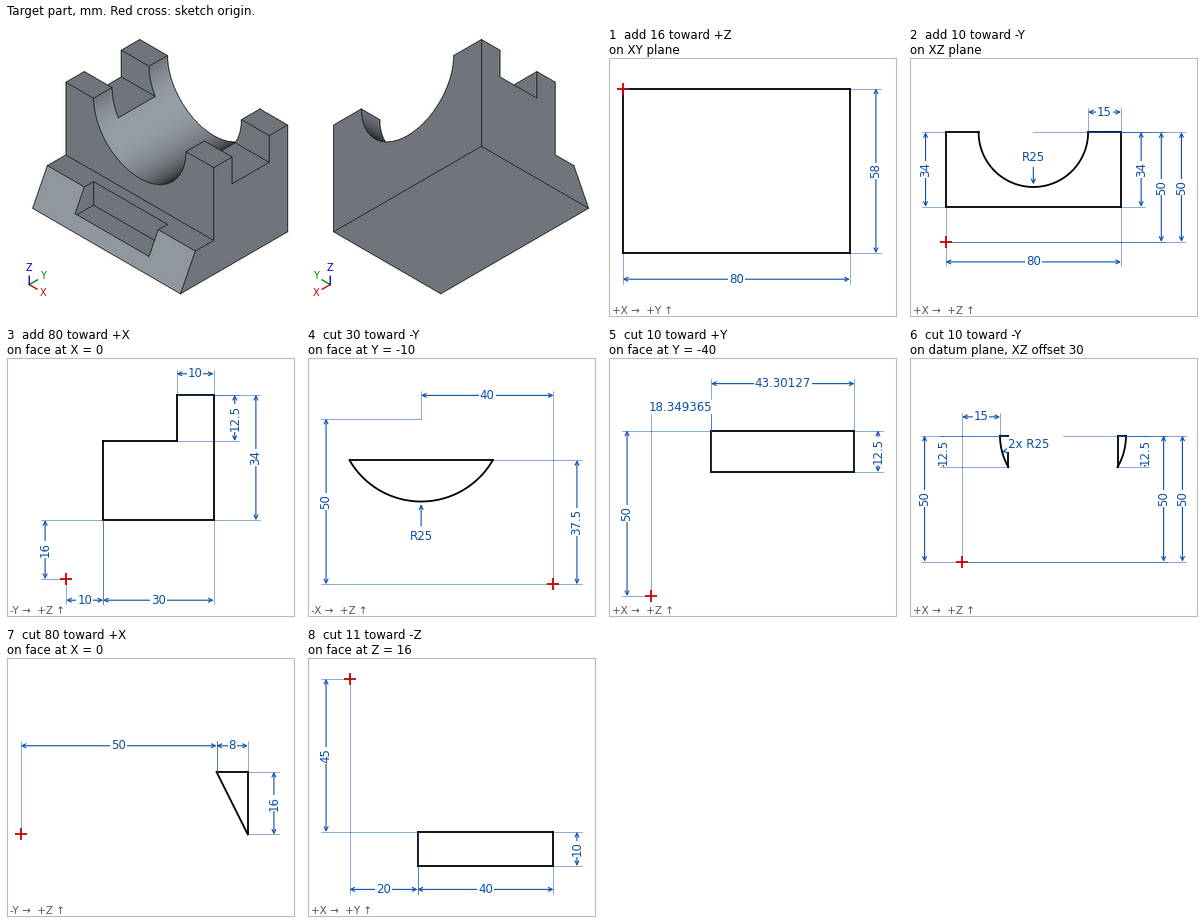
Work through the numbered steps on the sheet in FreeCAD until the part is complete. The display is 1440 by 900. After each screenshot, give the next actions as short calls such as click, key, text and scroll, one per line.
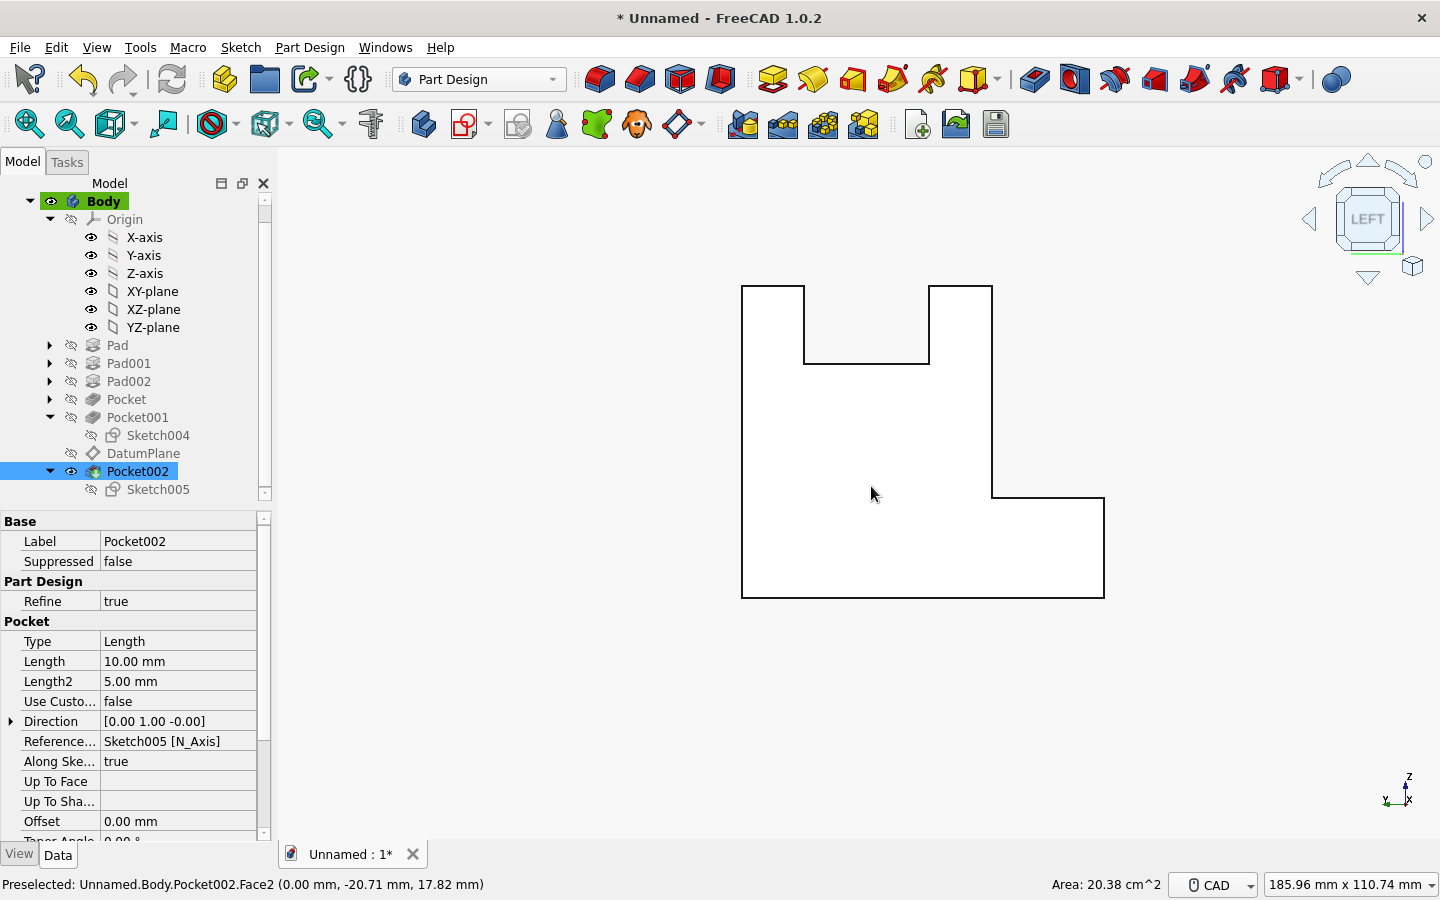
click(464, 124)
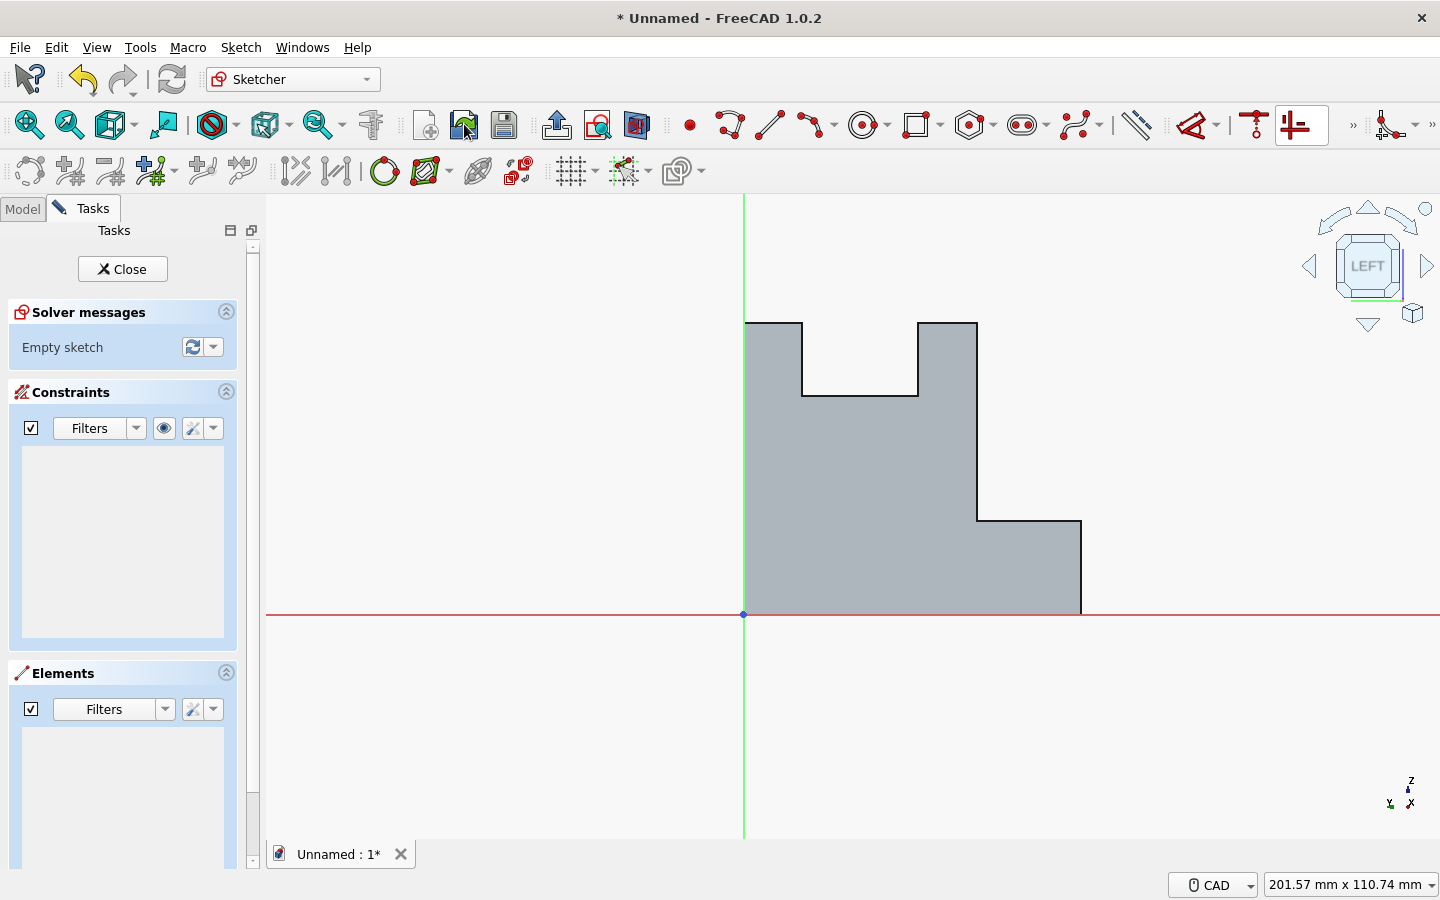
scroll(1148, 585, up, 7)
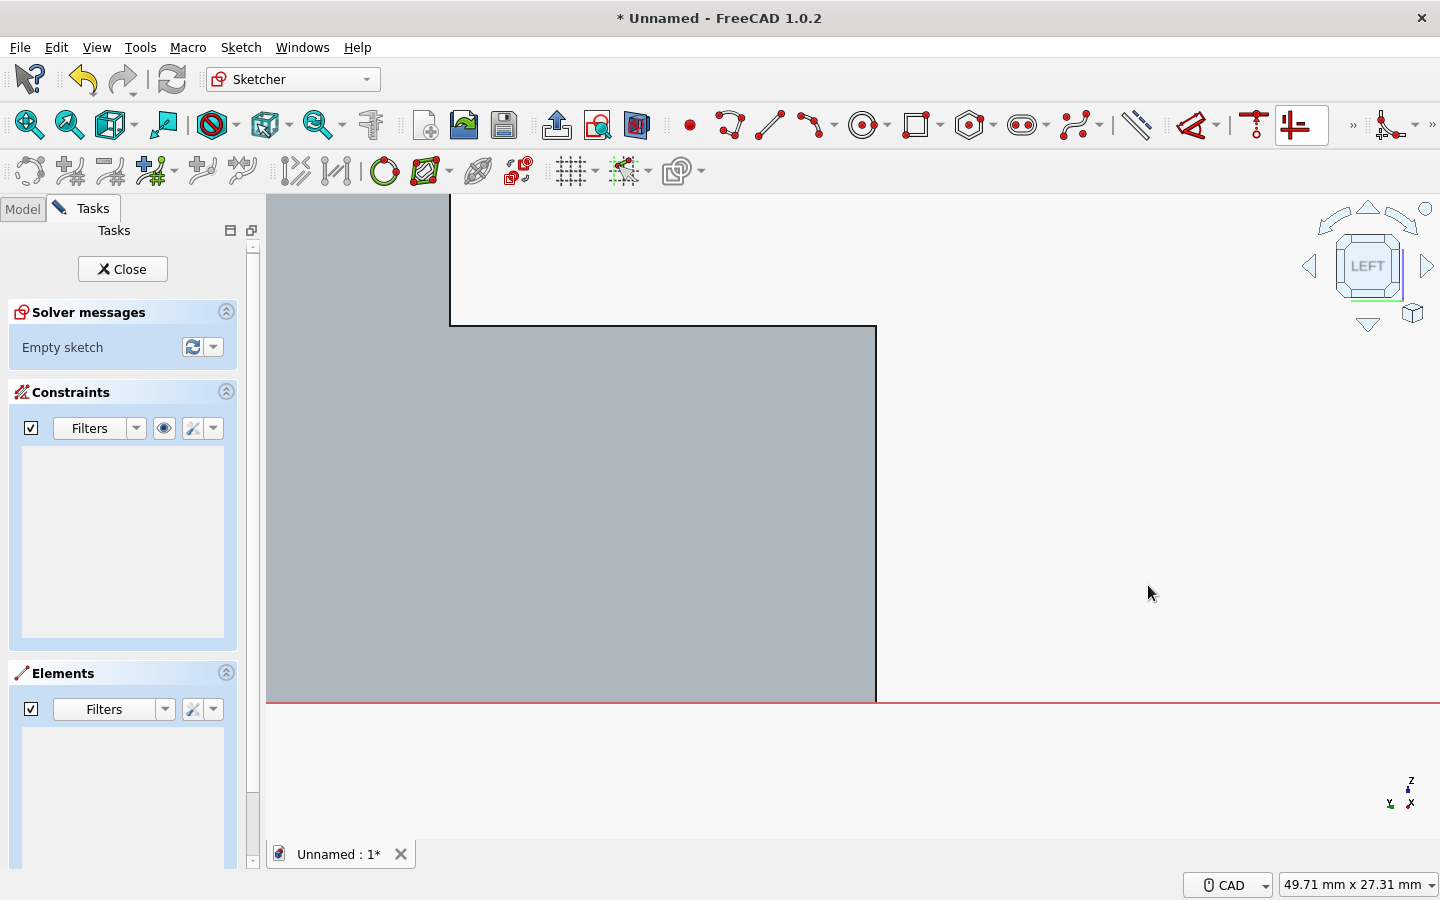
click(730, 126)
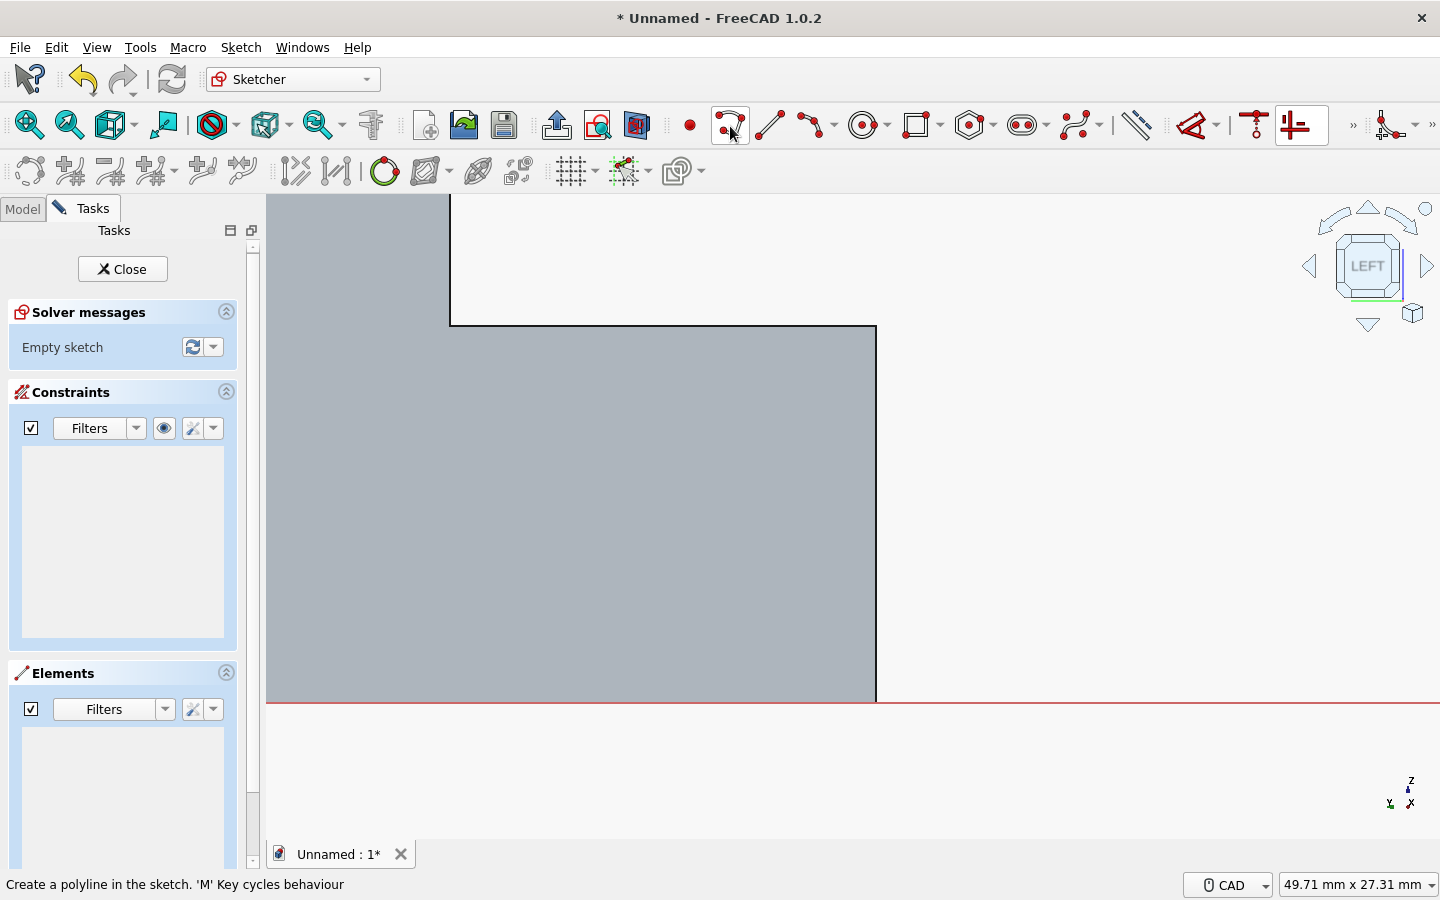
click(687, 326)
click(876, 703)
click(876, 326)
click(687, 327)
key(Escape)
key(Escape)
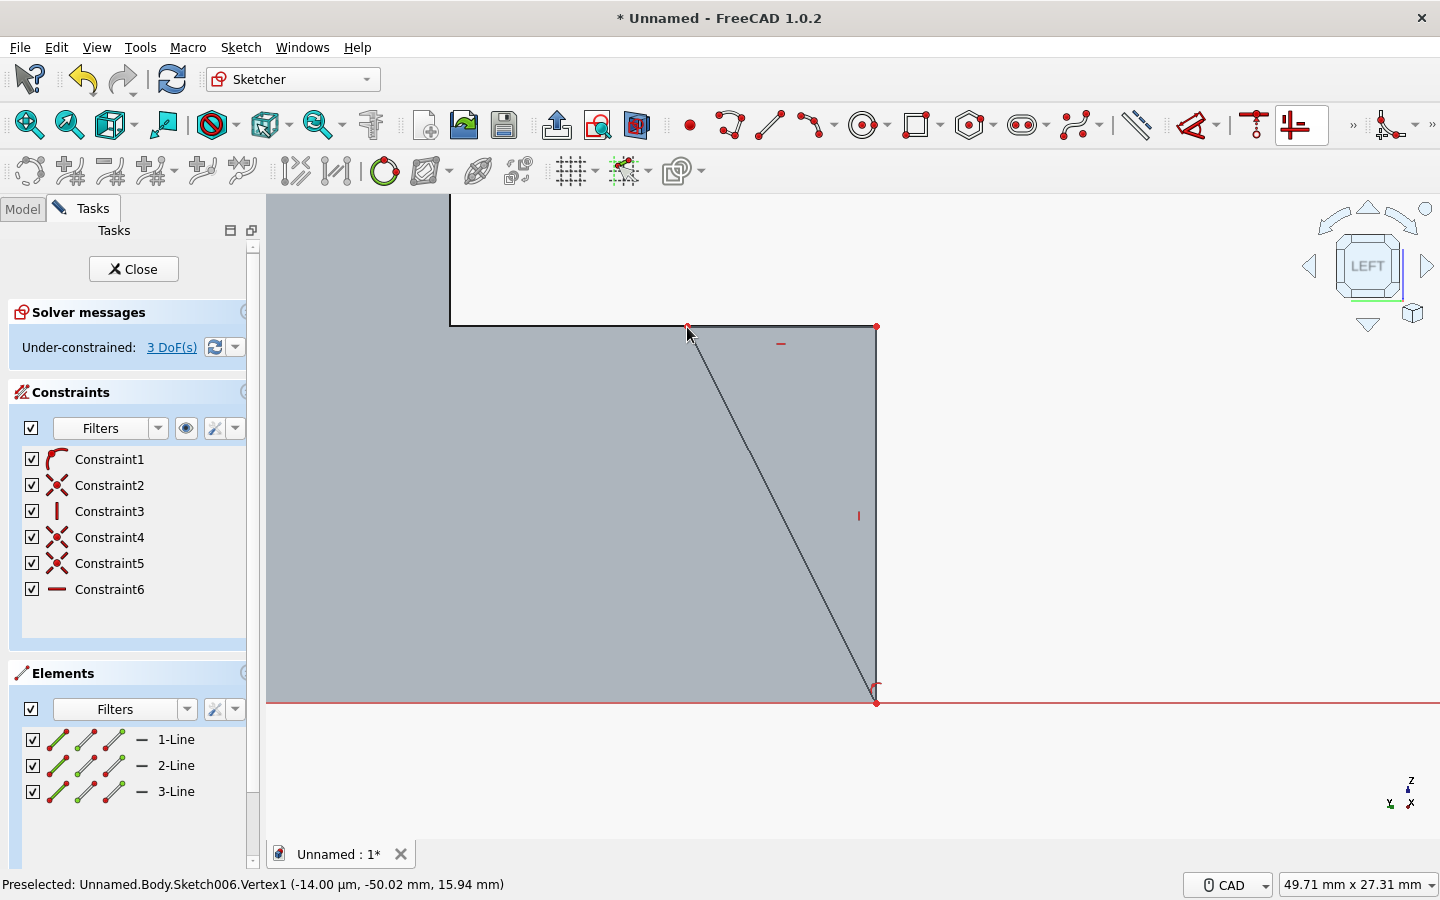
click(1192, 126)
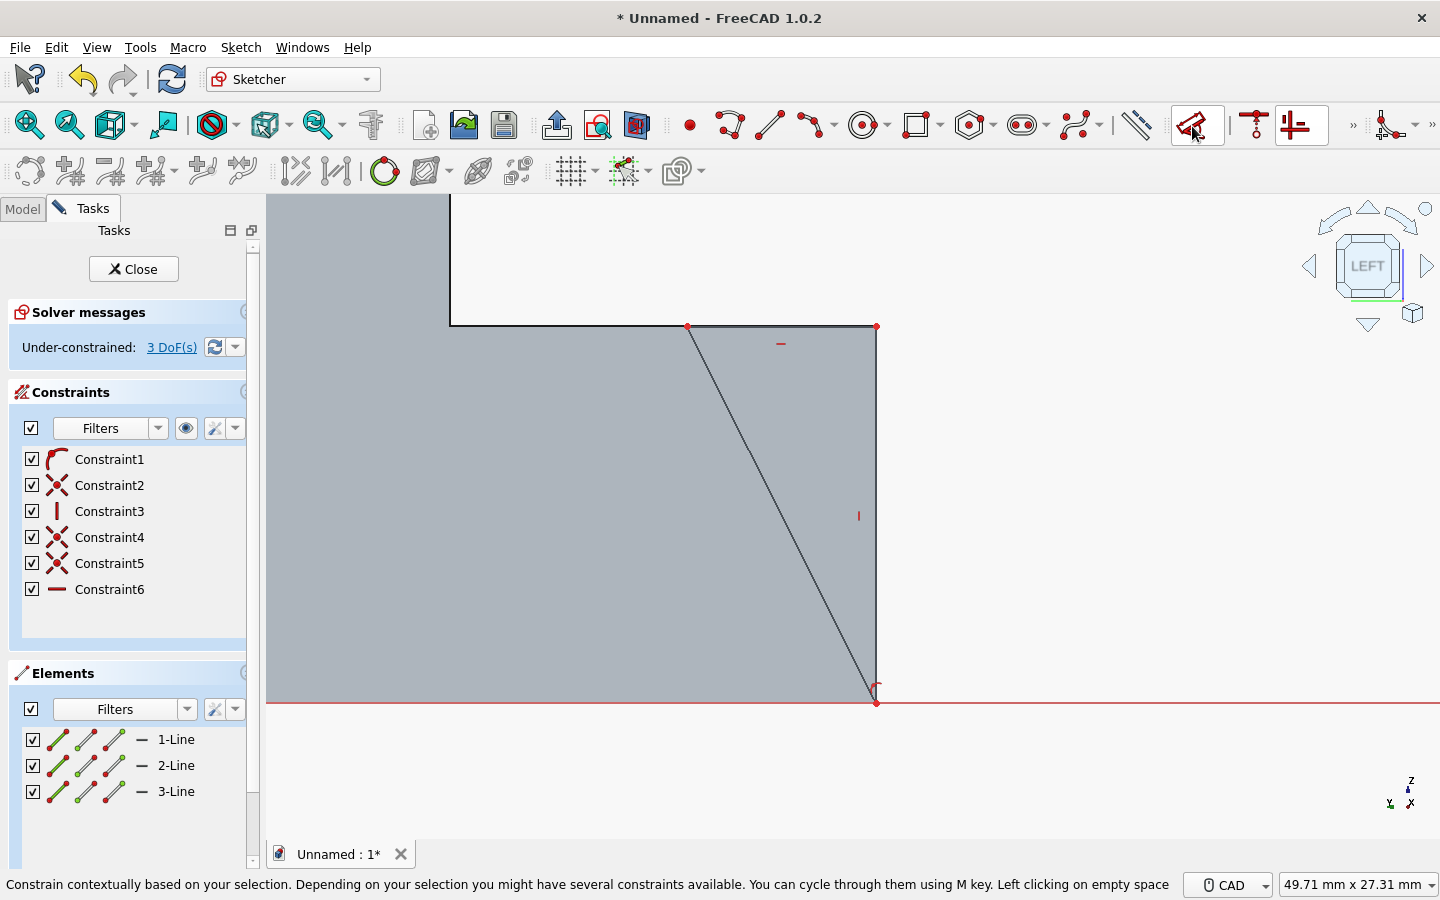
click(819, 327)
click(781, 293)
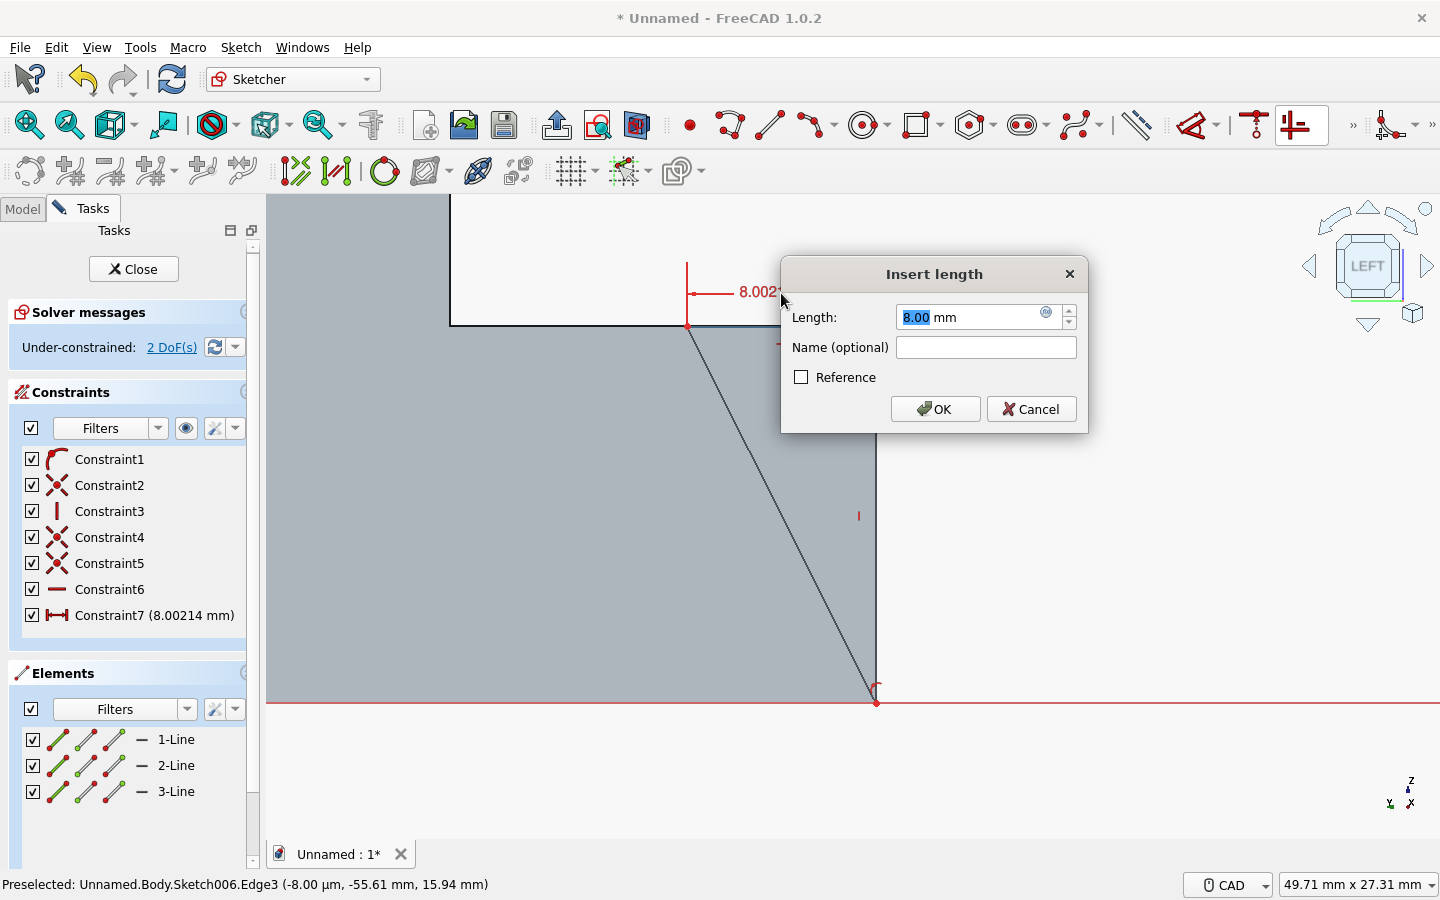
text(8)
key(Return)